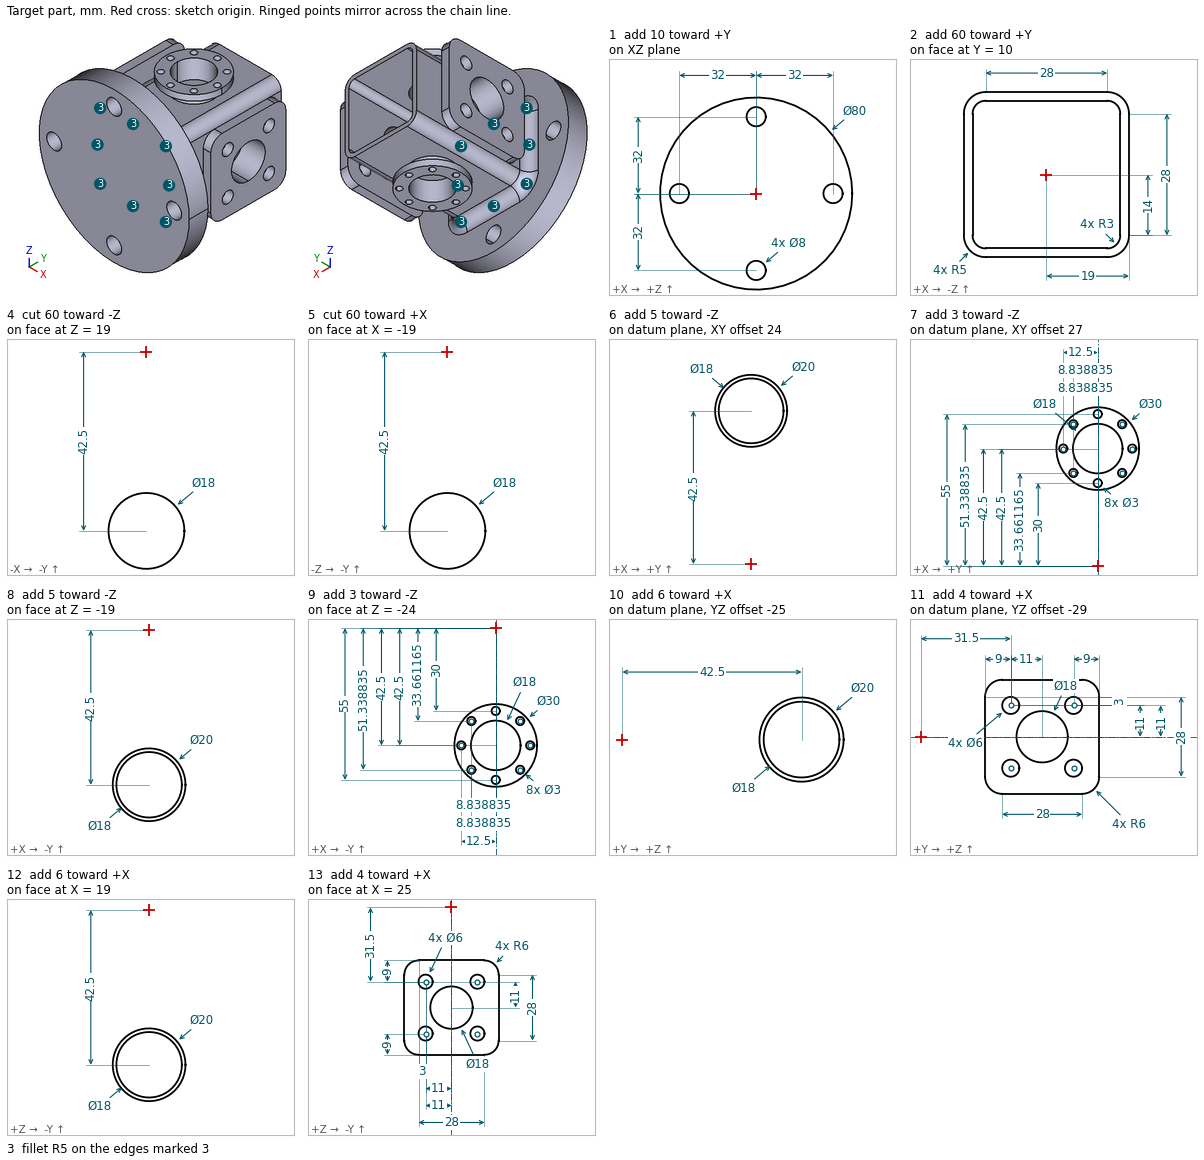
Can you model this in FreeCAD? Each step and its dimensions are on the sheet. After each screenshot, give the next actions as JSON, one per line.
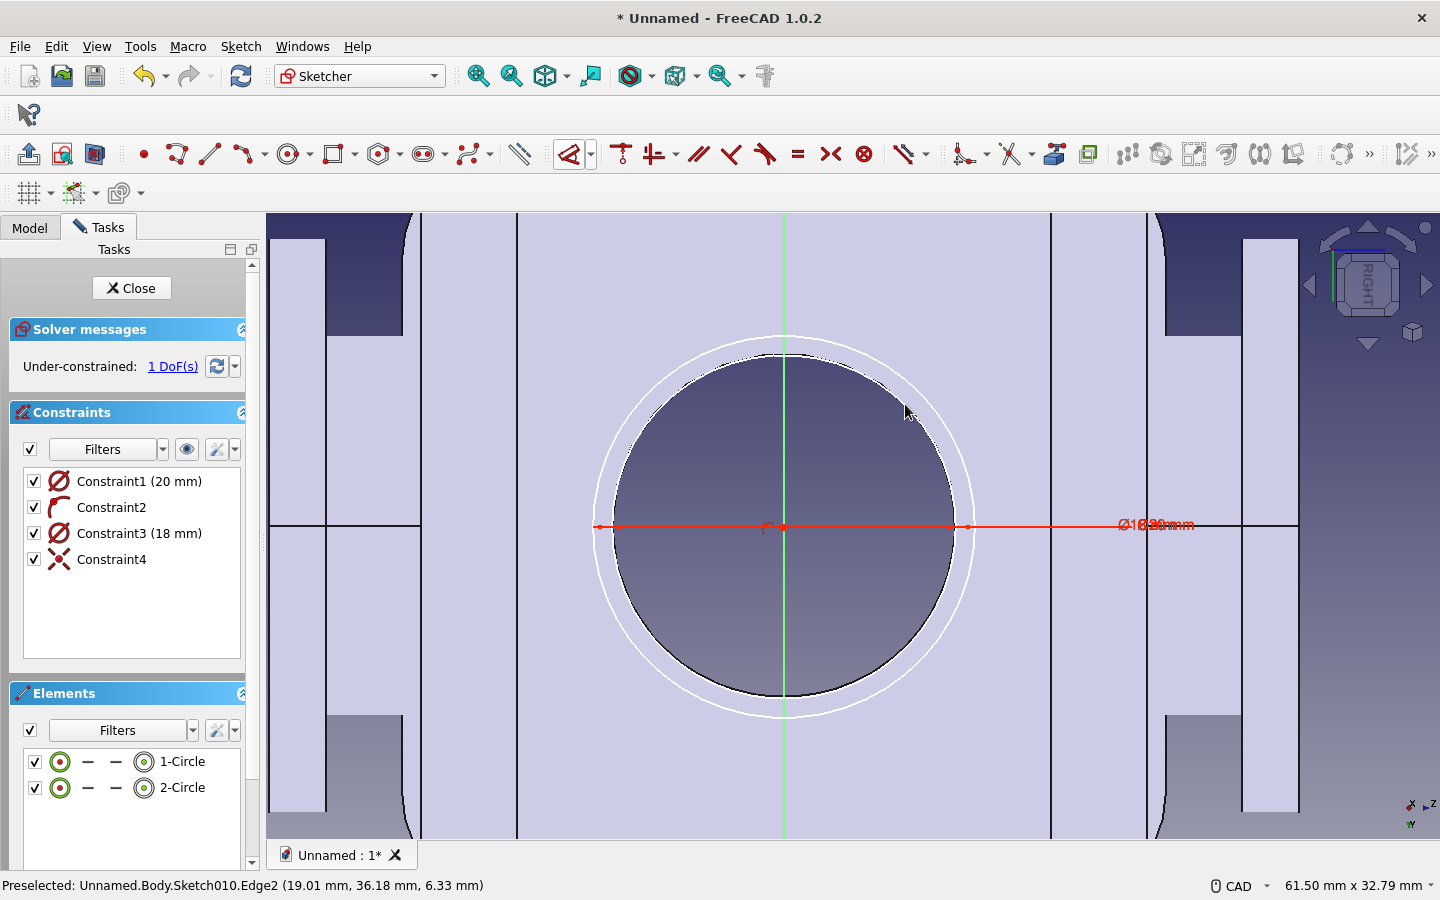
{"action": "left_click", "coordinate": [784, 527]}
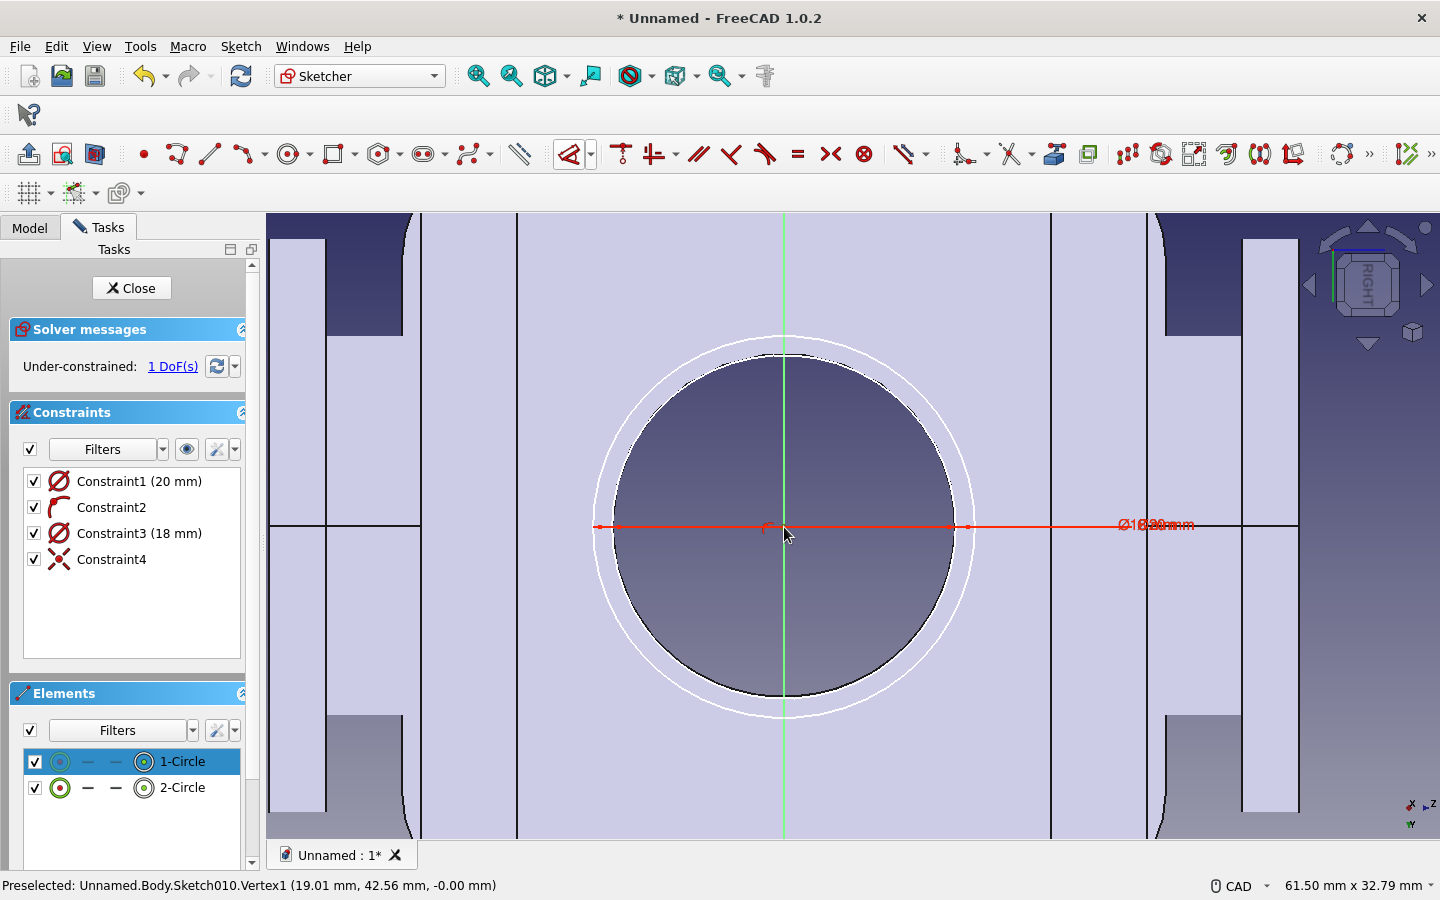
{"action": "key", "text": "i"}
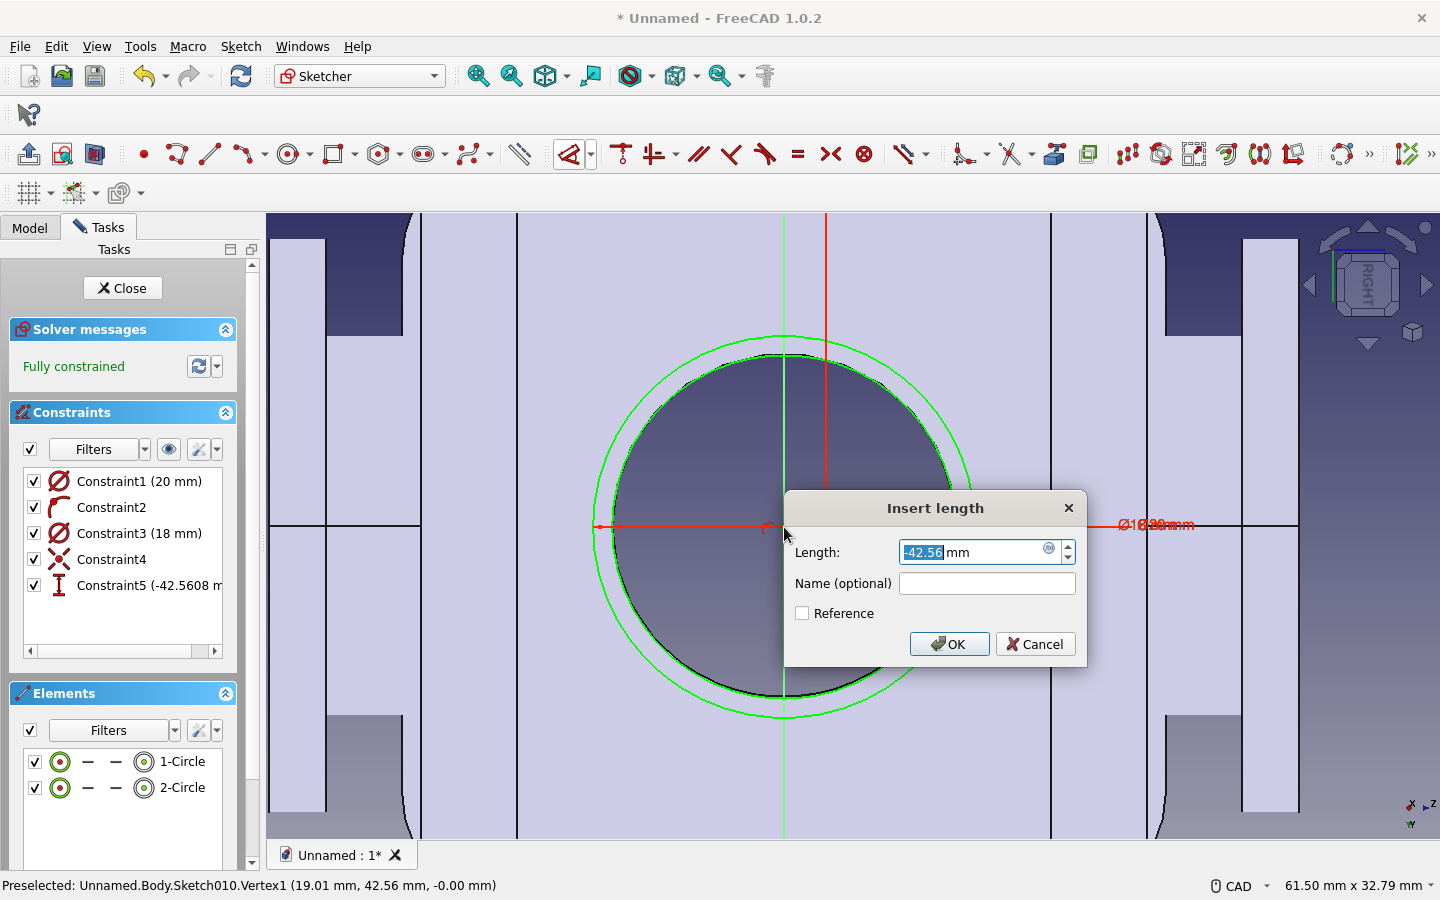
{"action": "type", "text": "-42.5"}
{"action": "key", "text": "Return"}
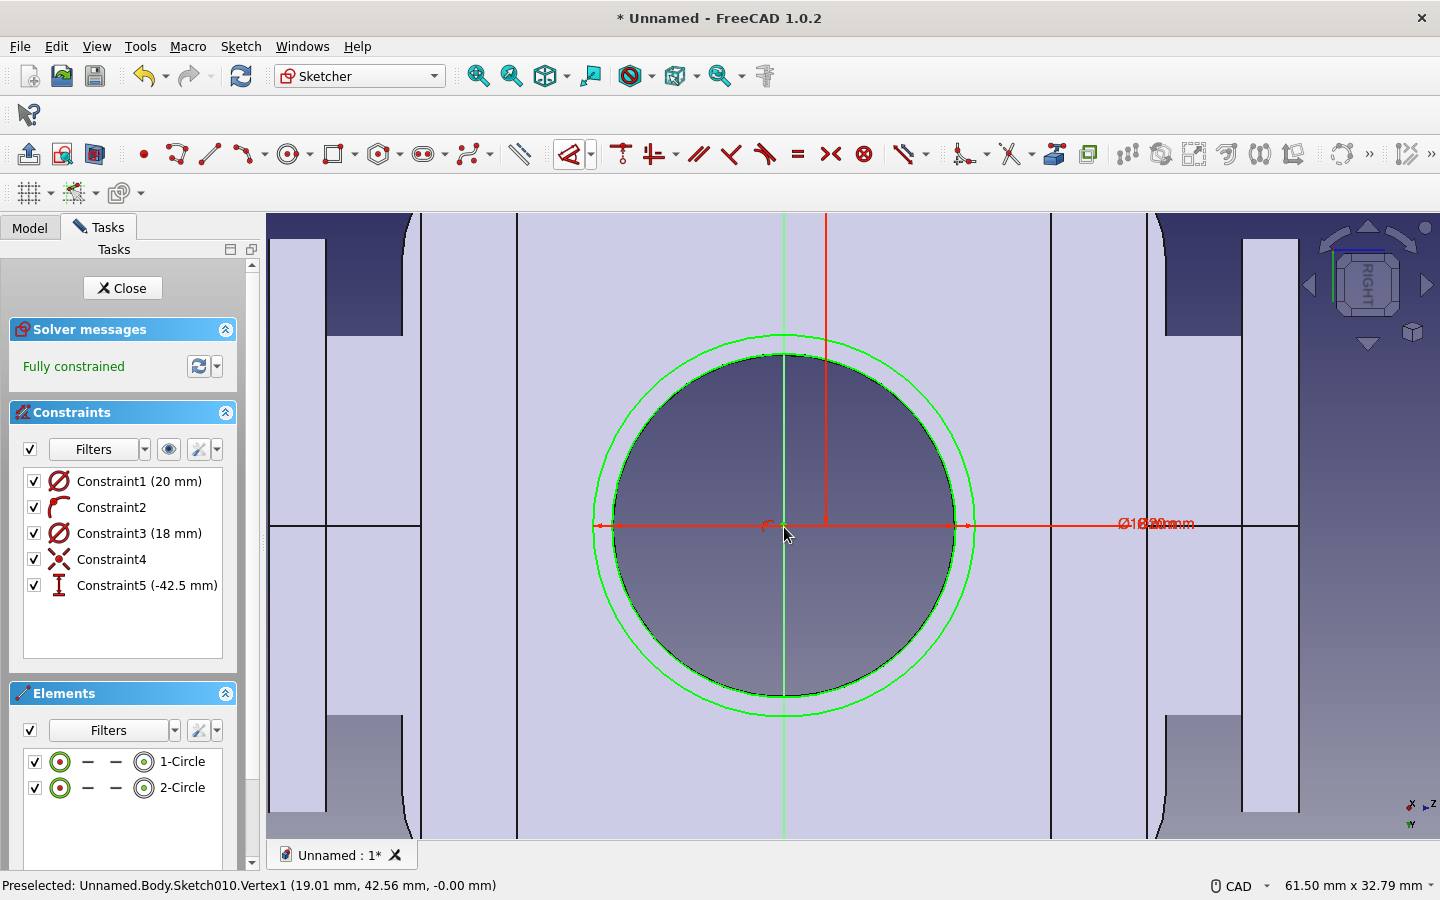
{"action": "left_click", "coordinate": [123, 288]}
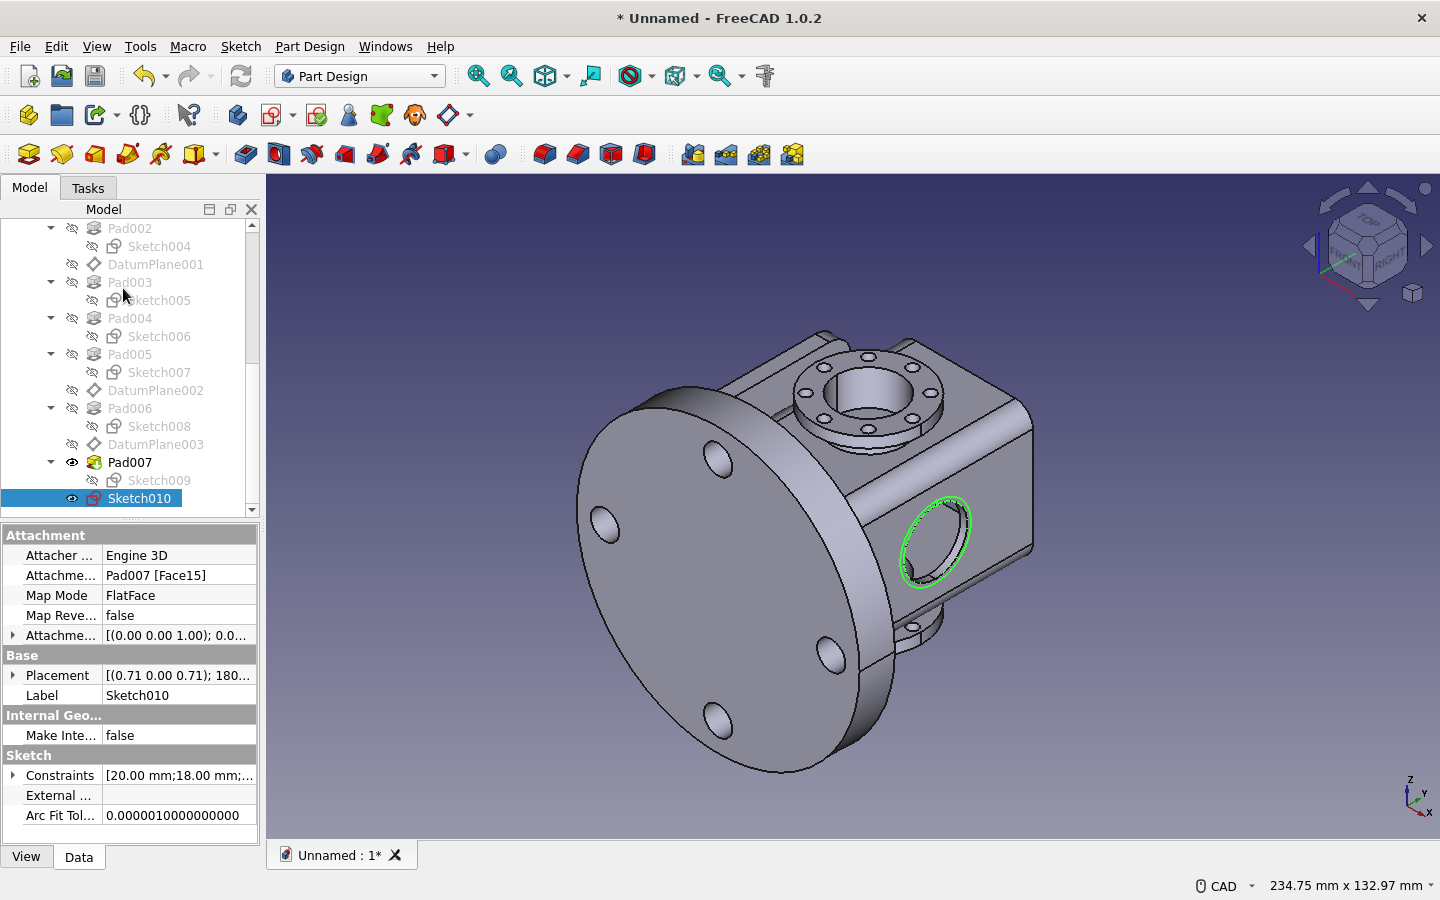
{"action": "left_click", "coordinate": [29, 154]}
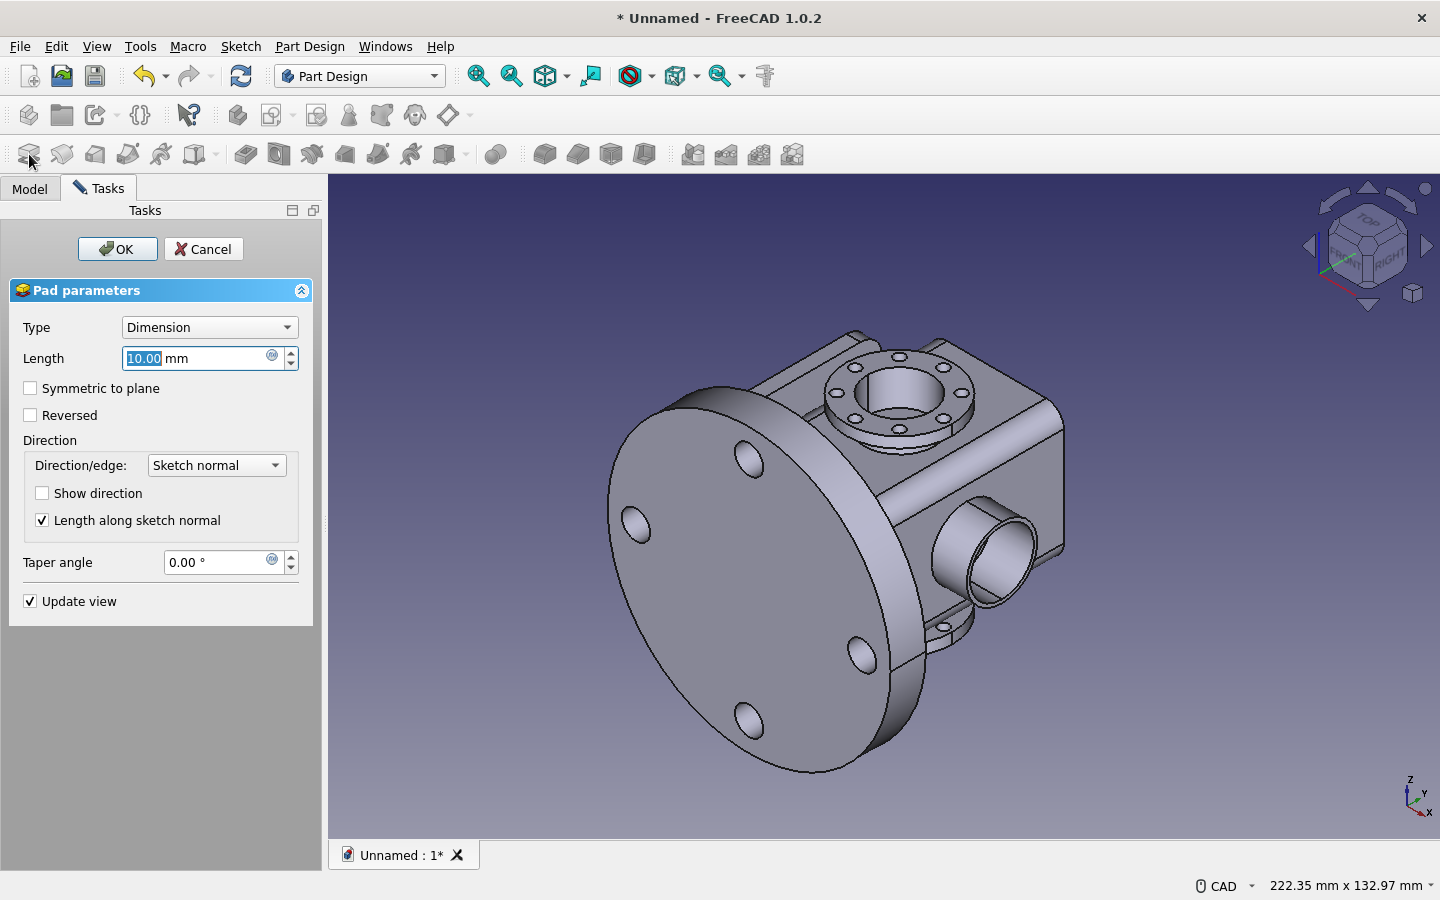
{"action": "type", "text": "6"}
{"action": "key", "text": "Tab"}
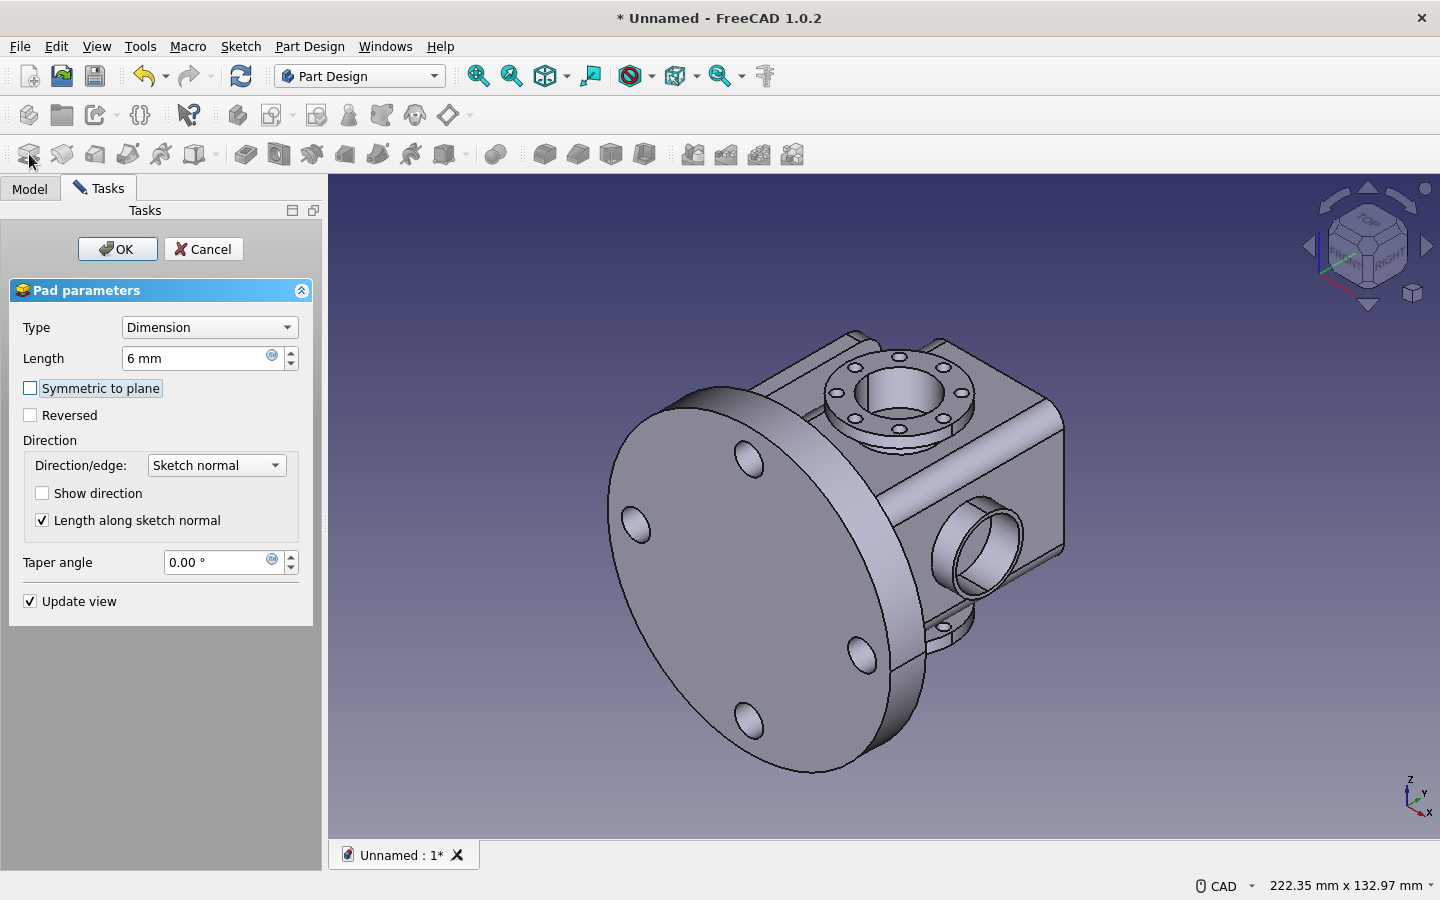
{"action": "left_click", "coordinate": [118, 249]}